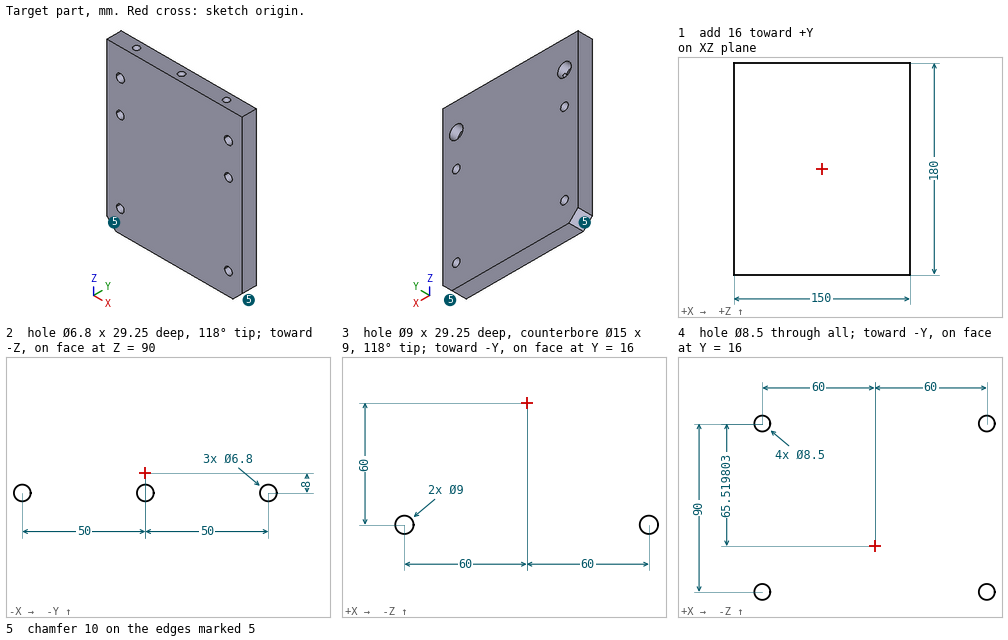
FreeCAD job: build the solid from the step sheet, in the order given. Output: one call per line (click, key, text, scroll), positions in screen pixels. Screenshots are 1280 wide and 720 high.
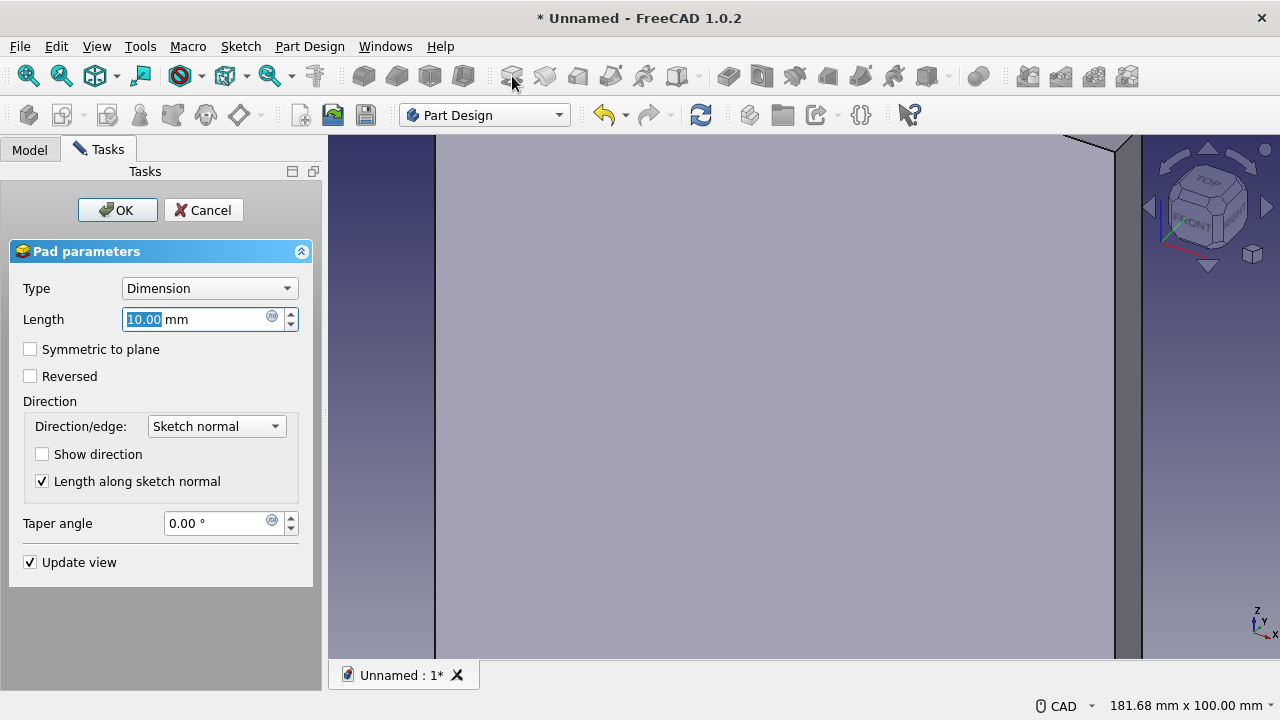
text(16)
key(Tab)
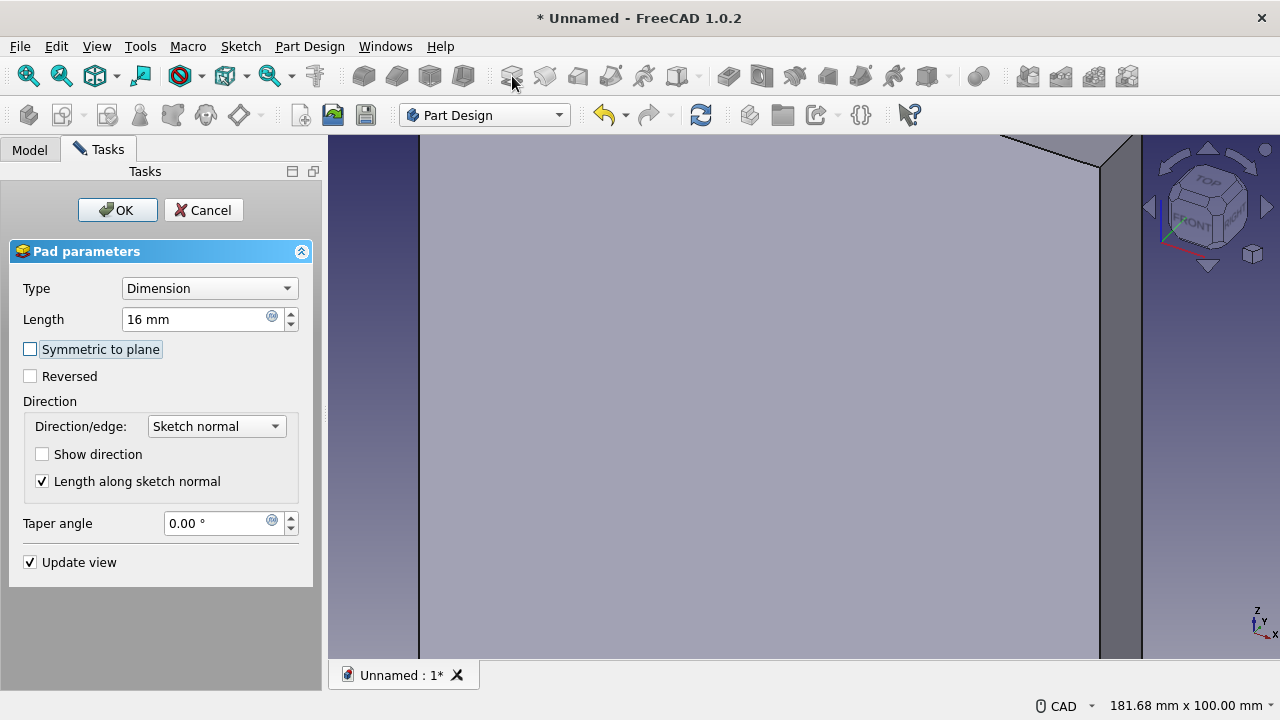
click(31, 376)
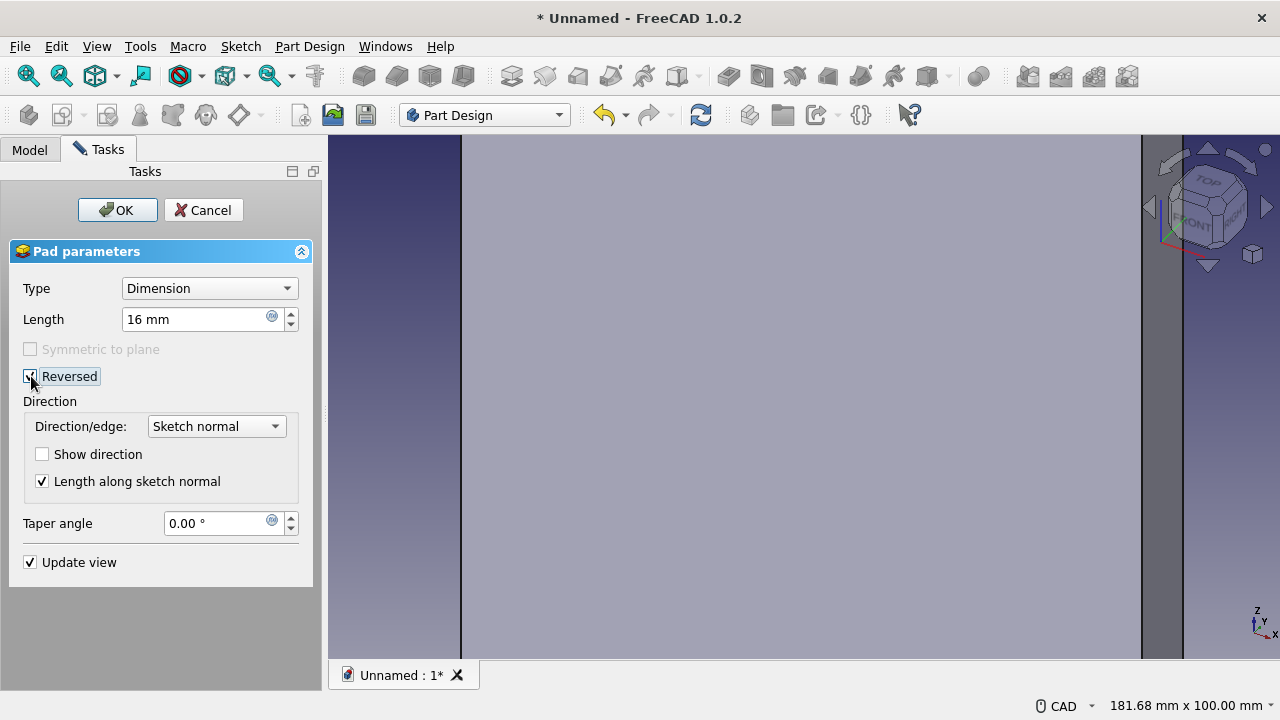
click(118, 210)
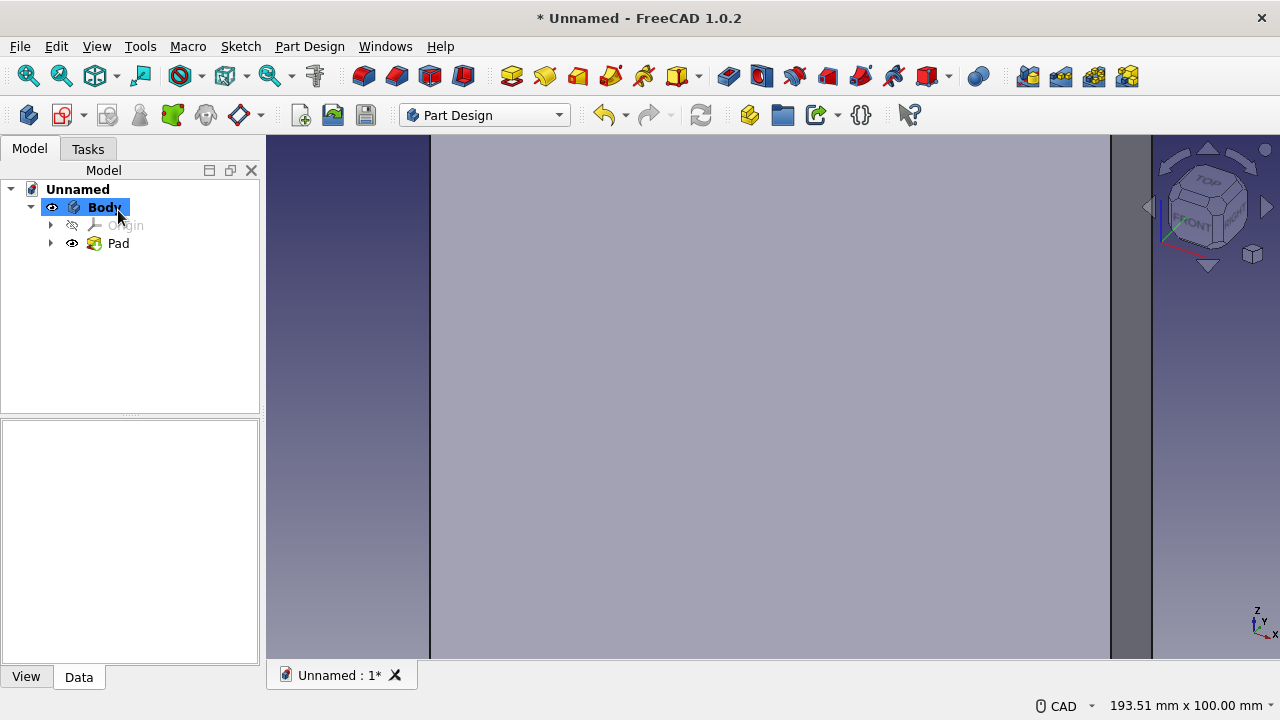
click(29, 76)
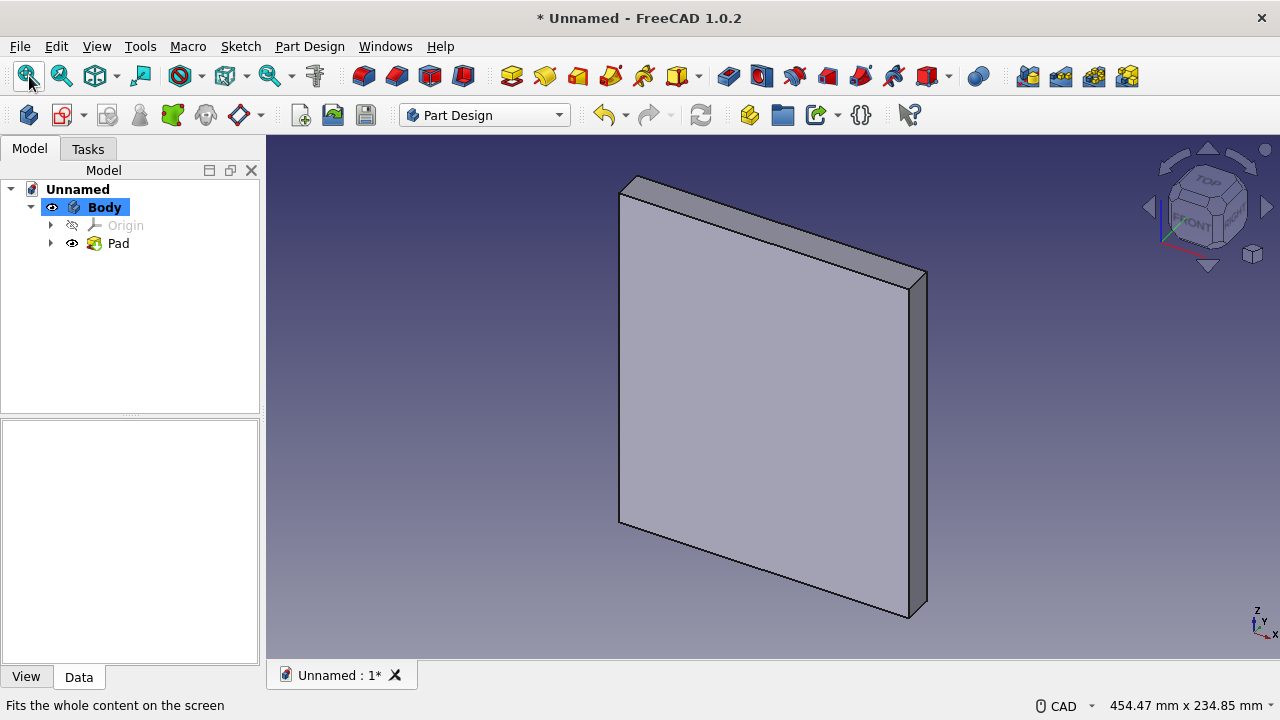
click(897, 273)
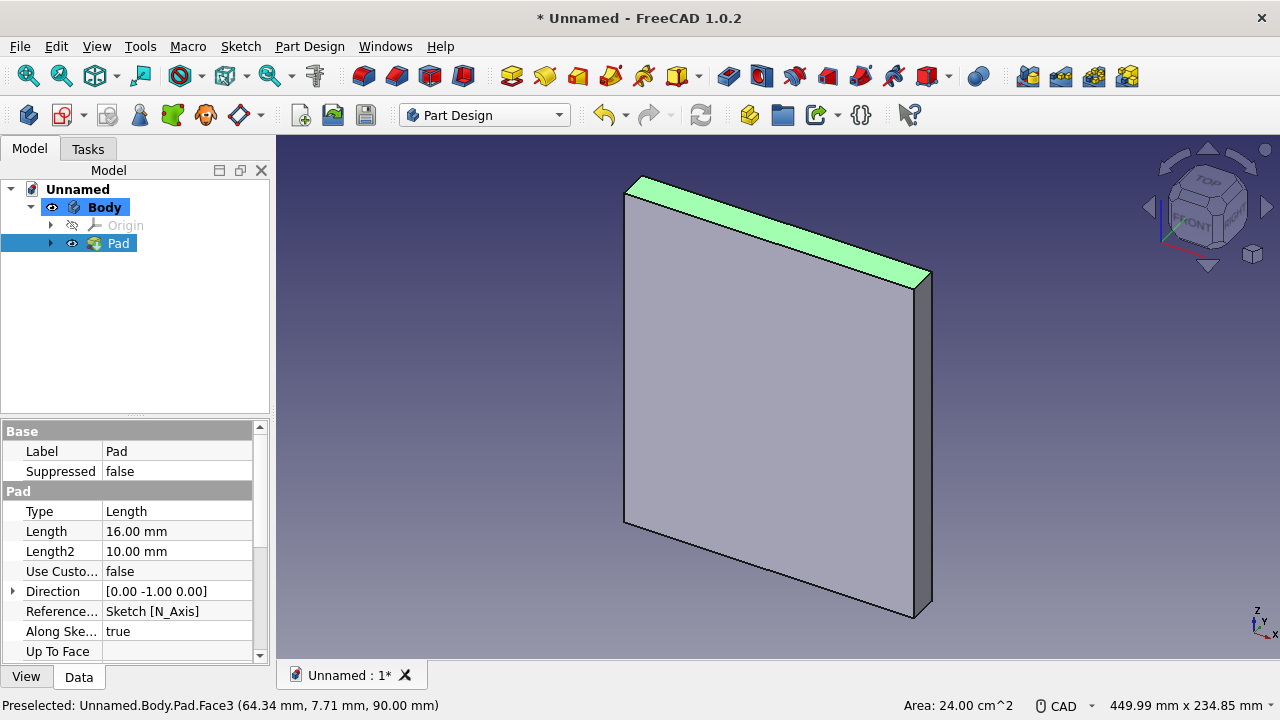
click(62, 116)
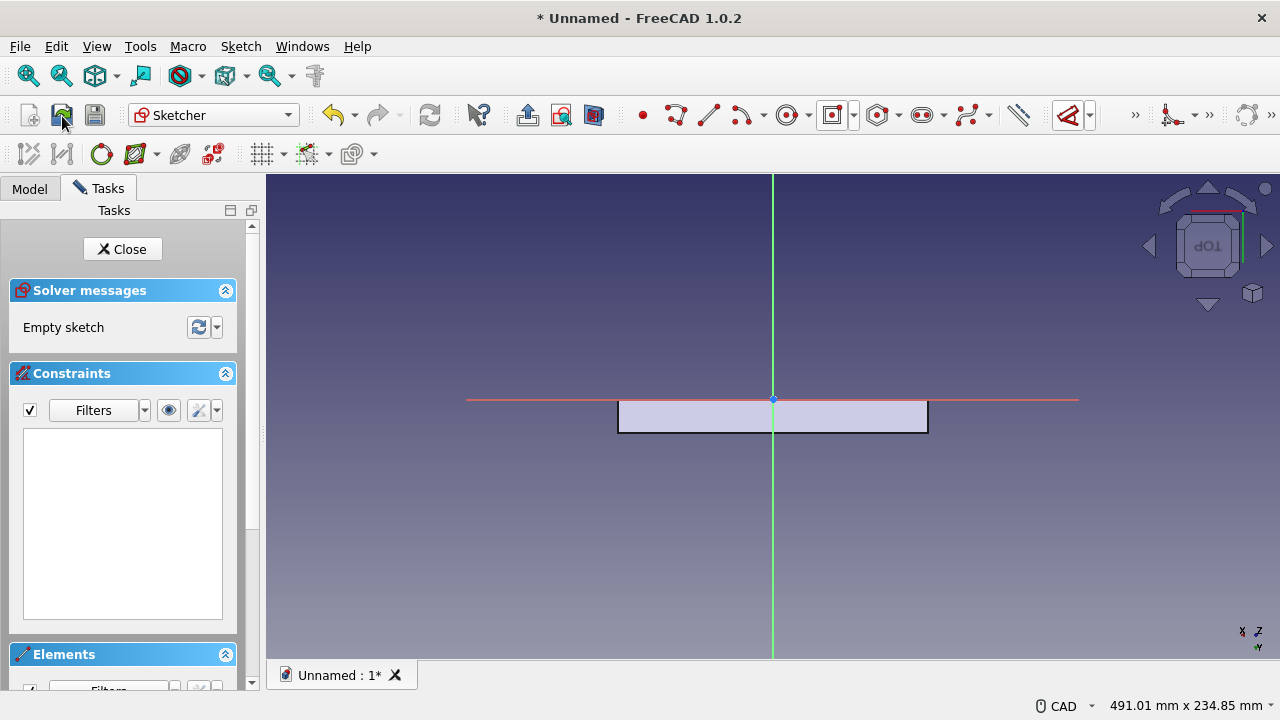
scroll(813, 409, up, 5)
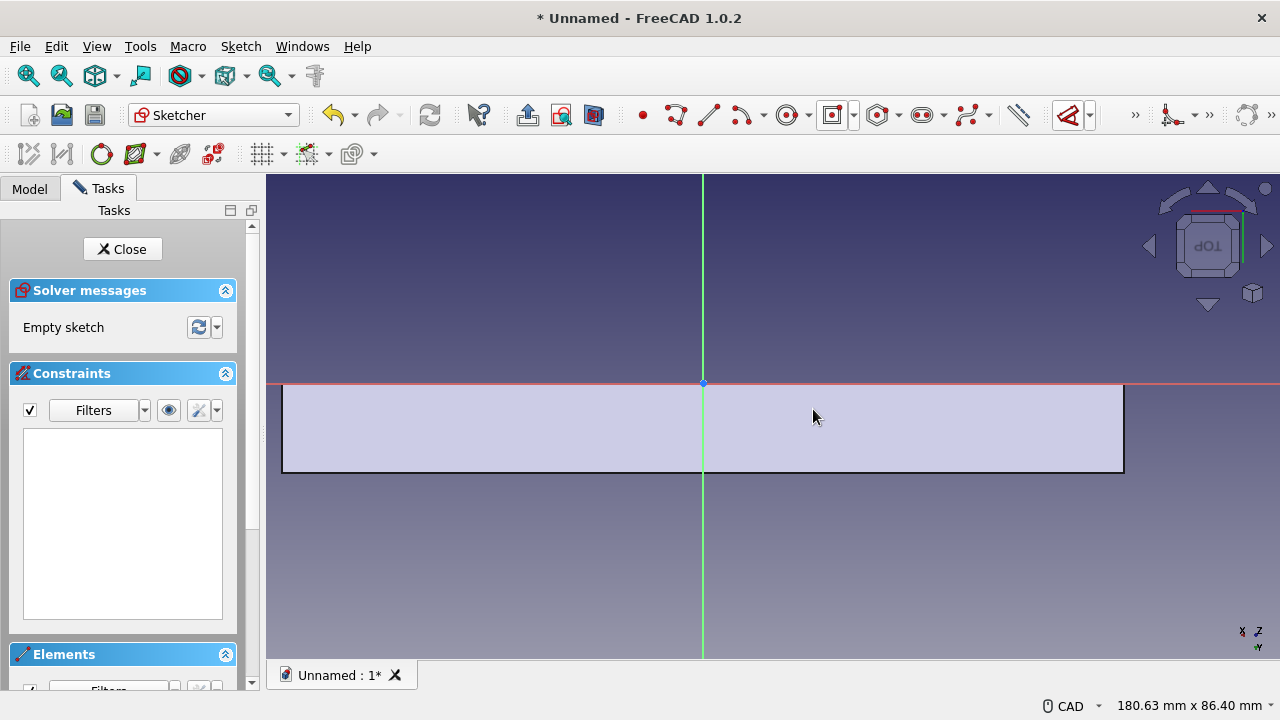
click(786, 116)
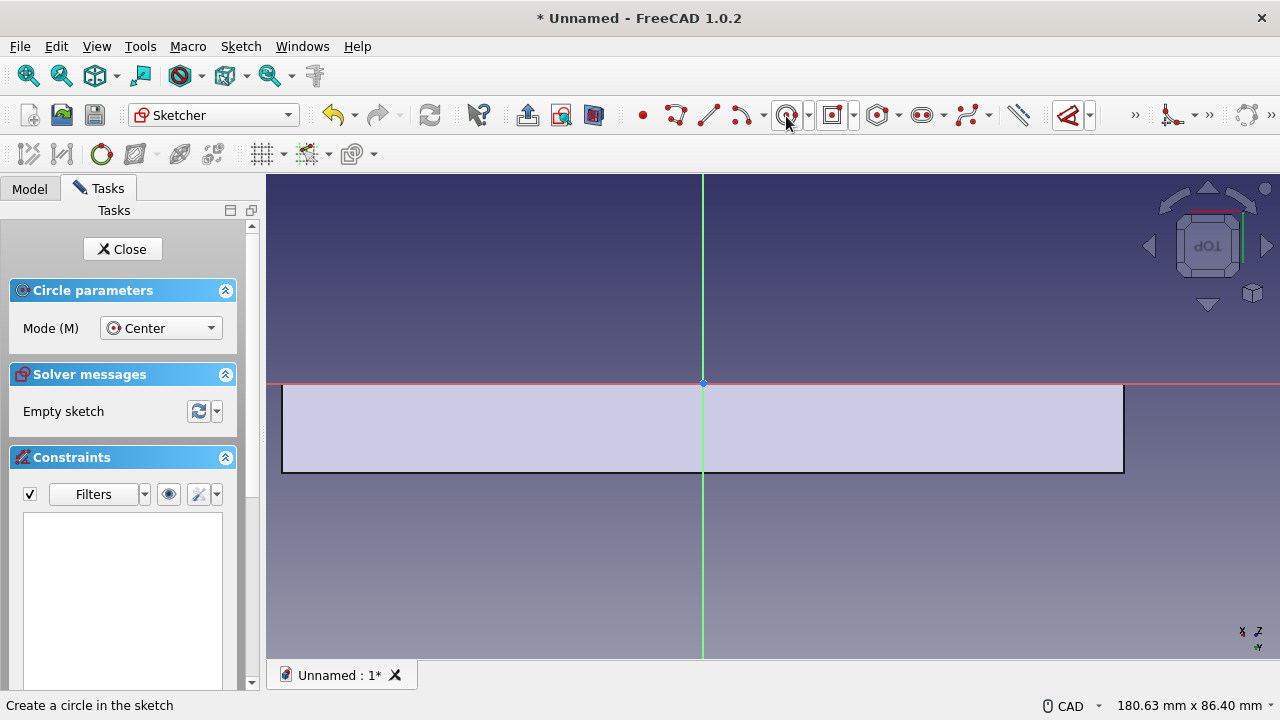
click(984, 429)
move(998, 415)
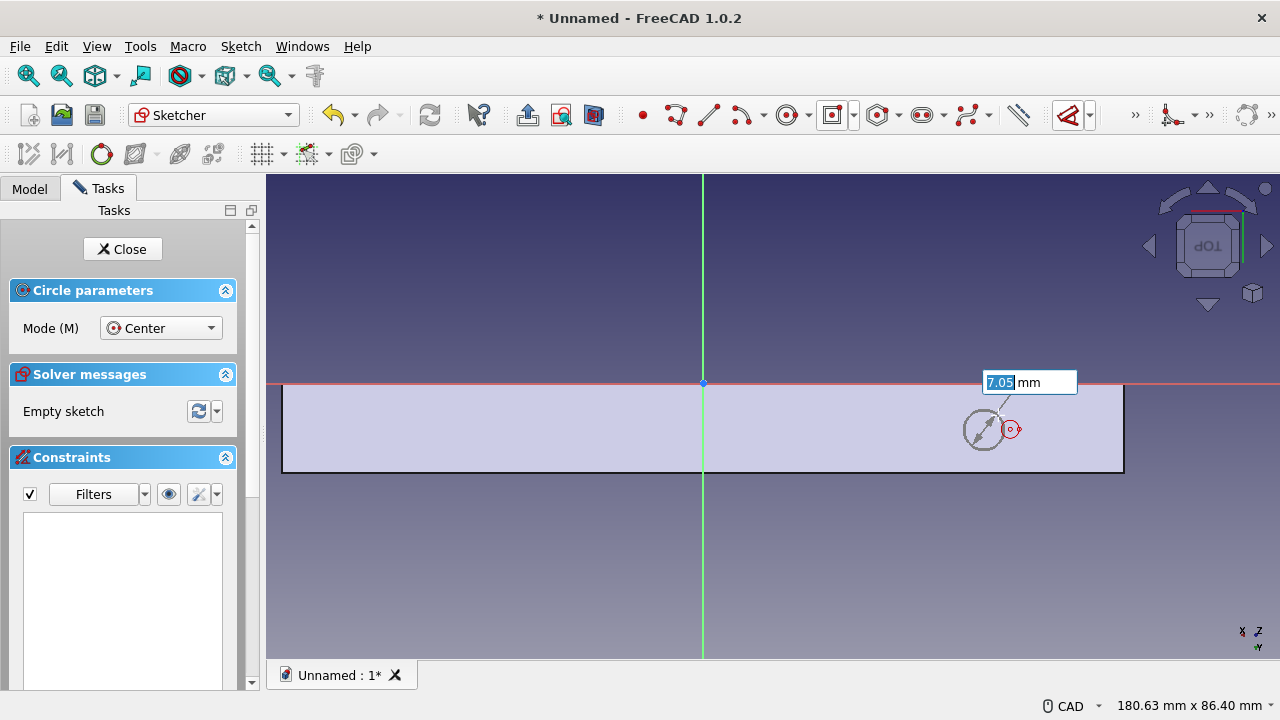
text(6.8)
key(Return)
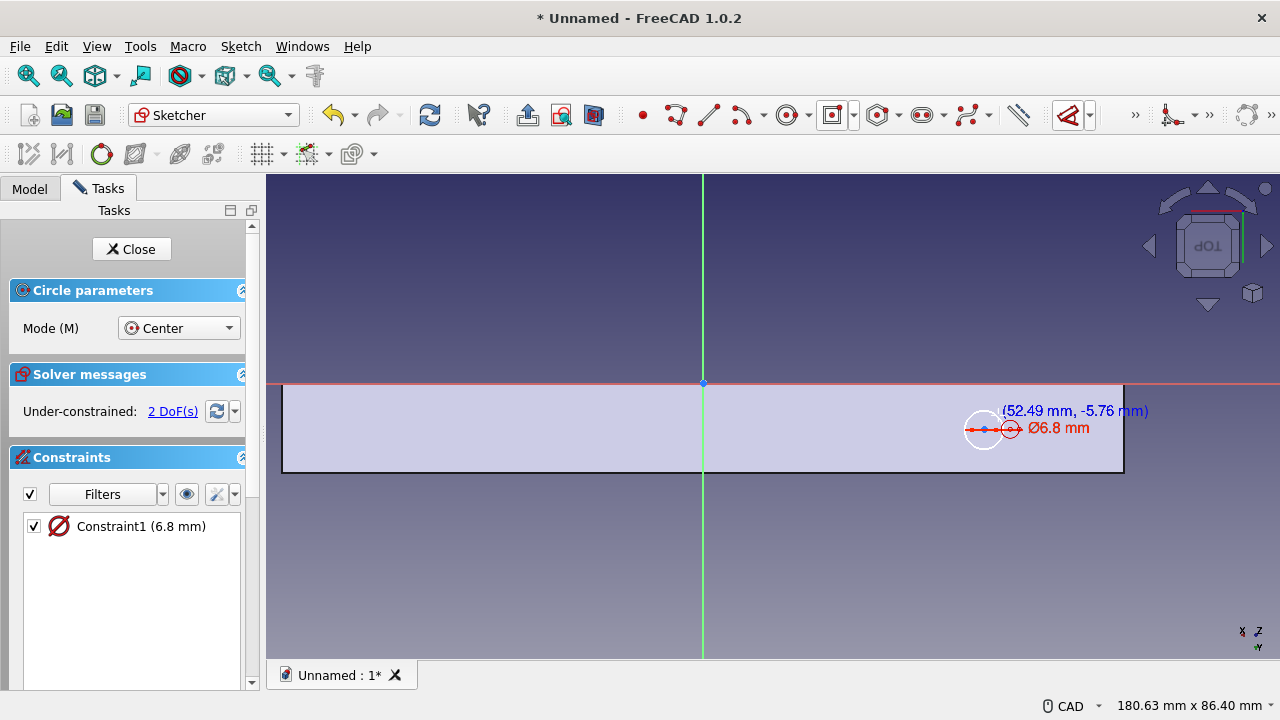
click(703, 429)
move(721, 422)